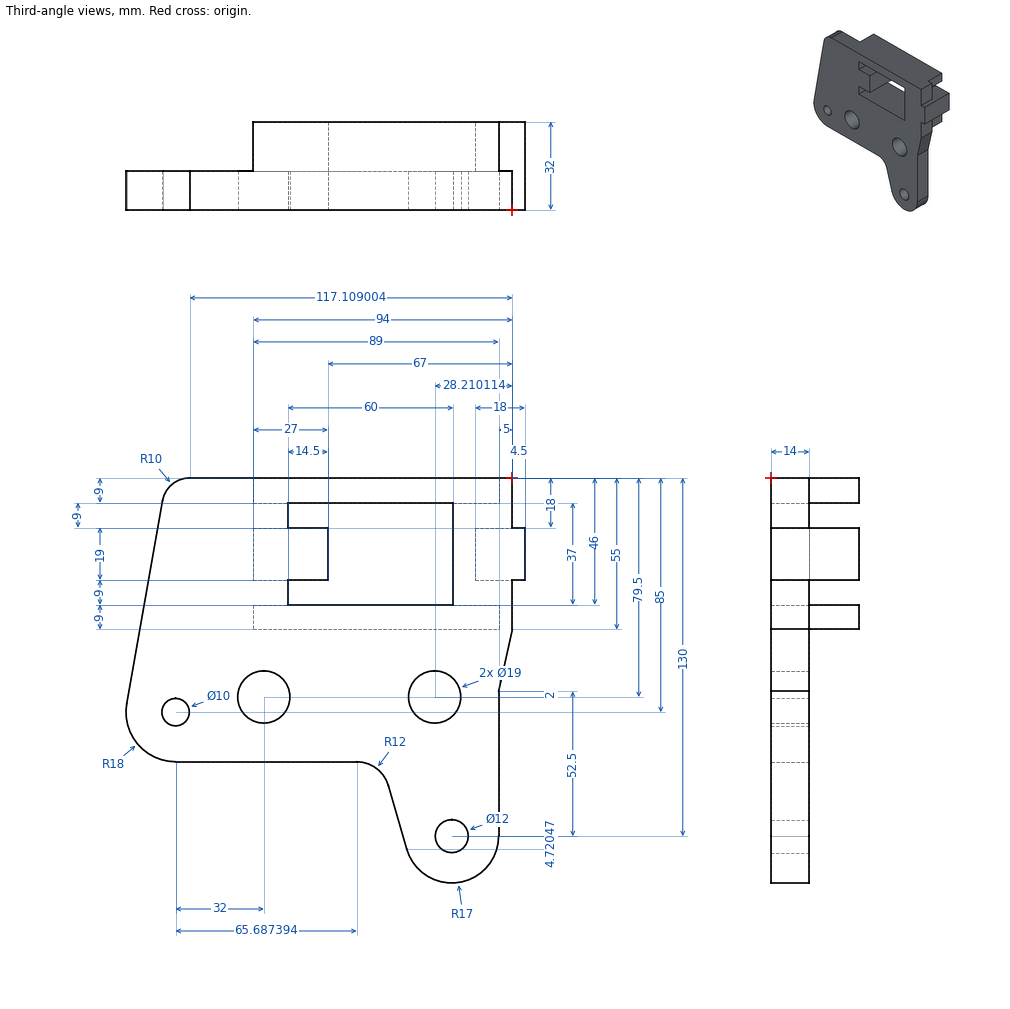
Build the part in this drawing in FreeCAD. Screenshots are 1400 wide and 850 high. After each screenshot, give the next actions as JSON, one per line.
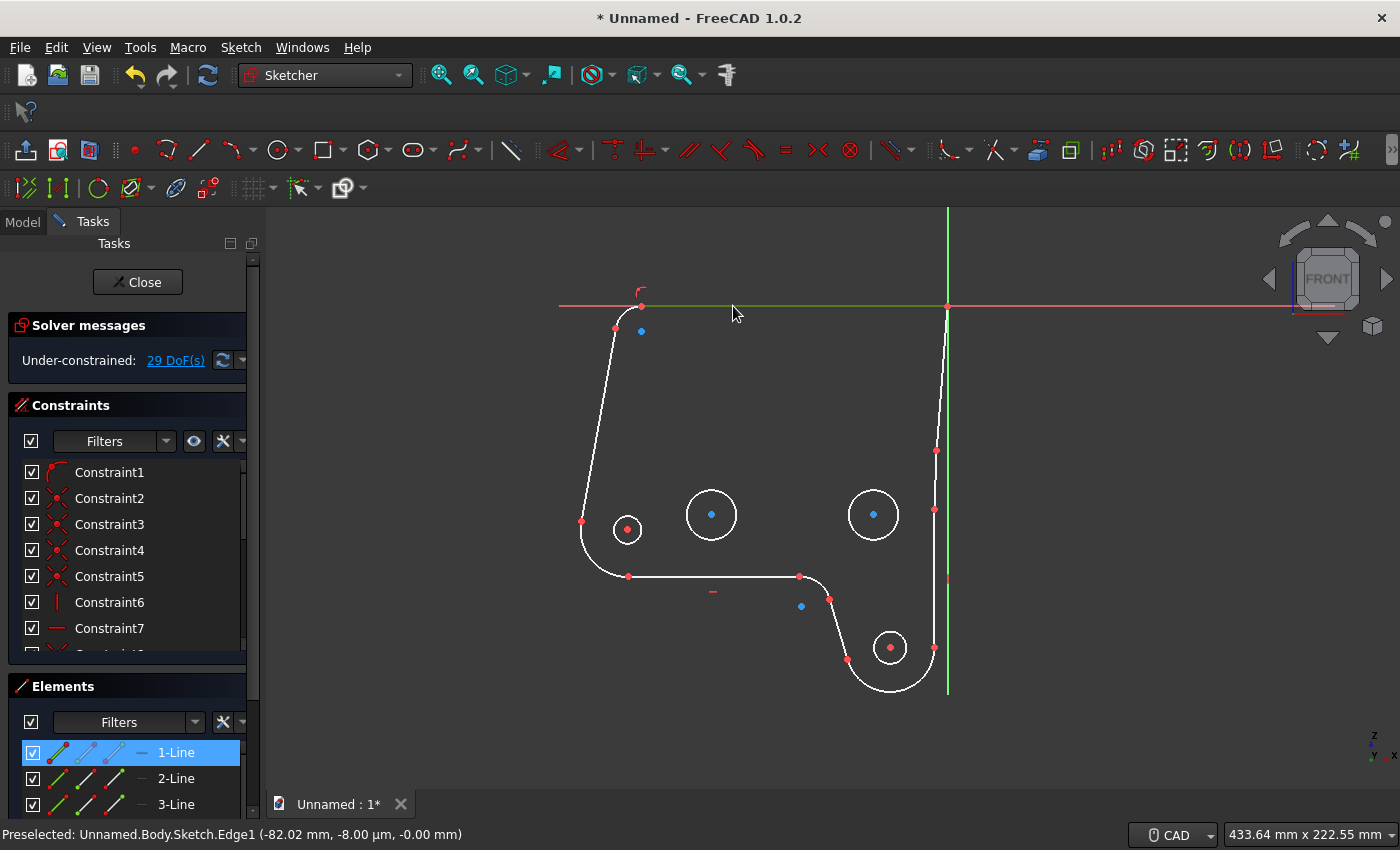
{"action": "scroll", "coordinate": [630, 309], "scroll_direction": "up", "scroll_amount": 2}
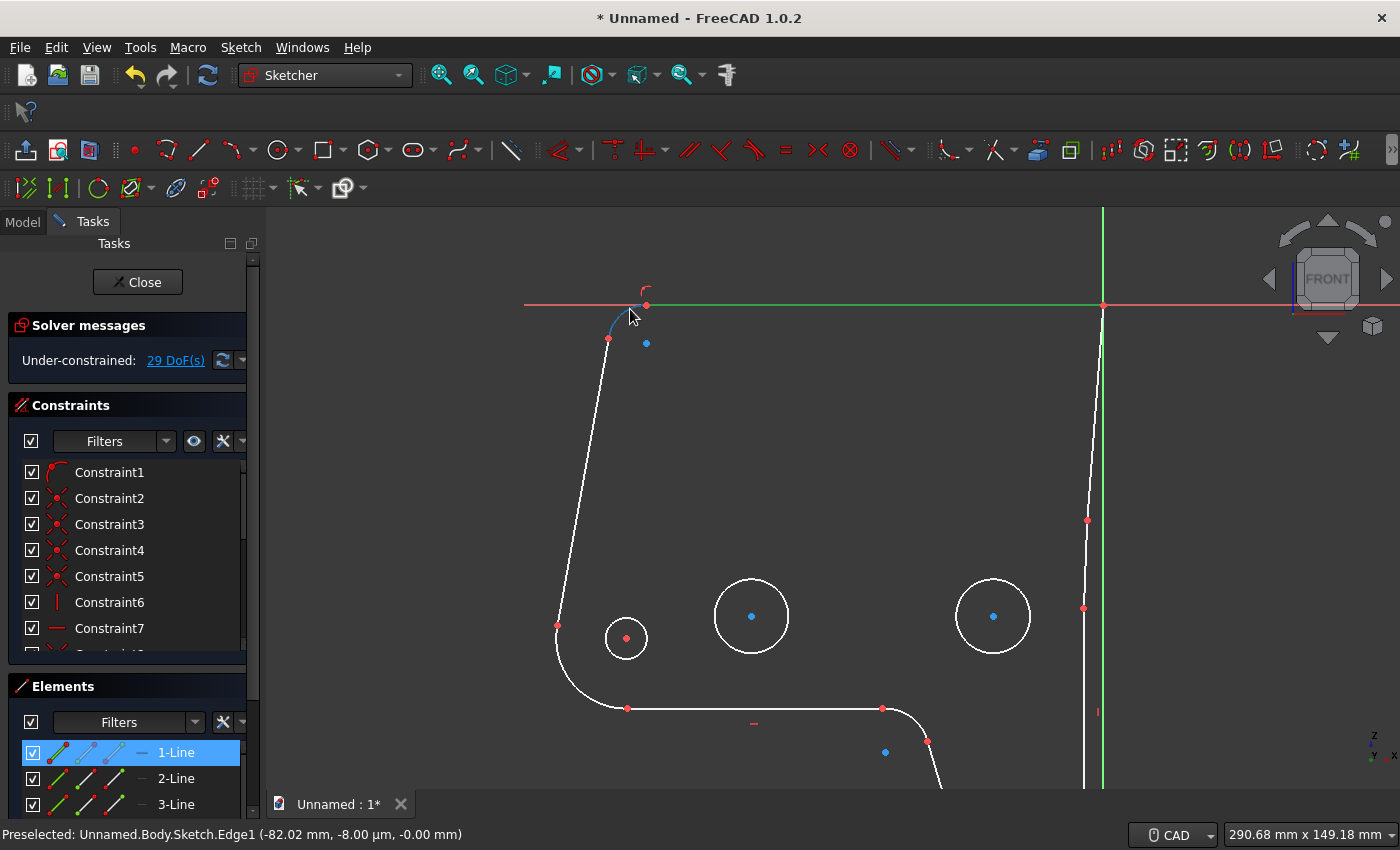
{"action": "left_click", "coordinate": [630, 309]}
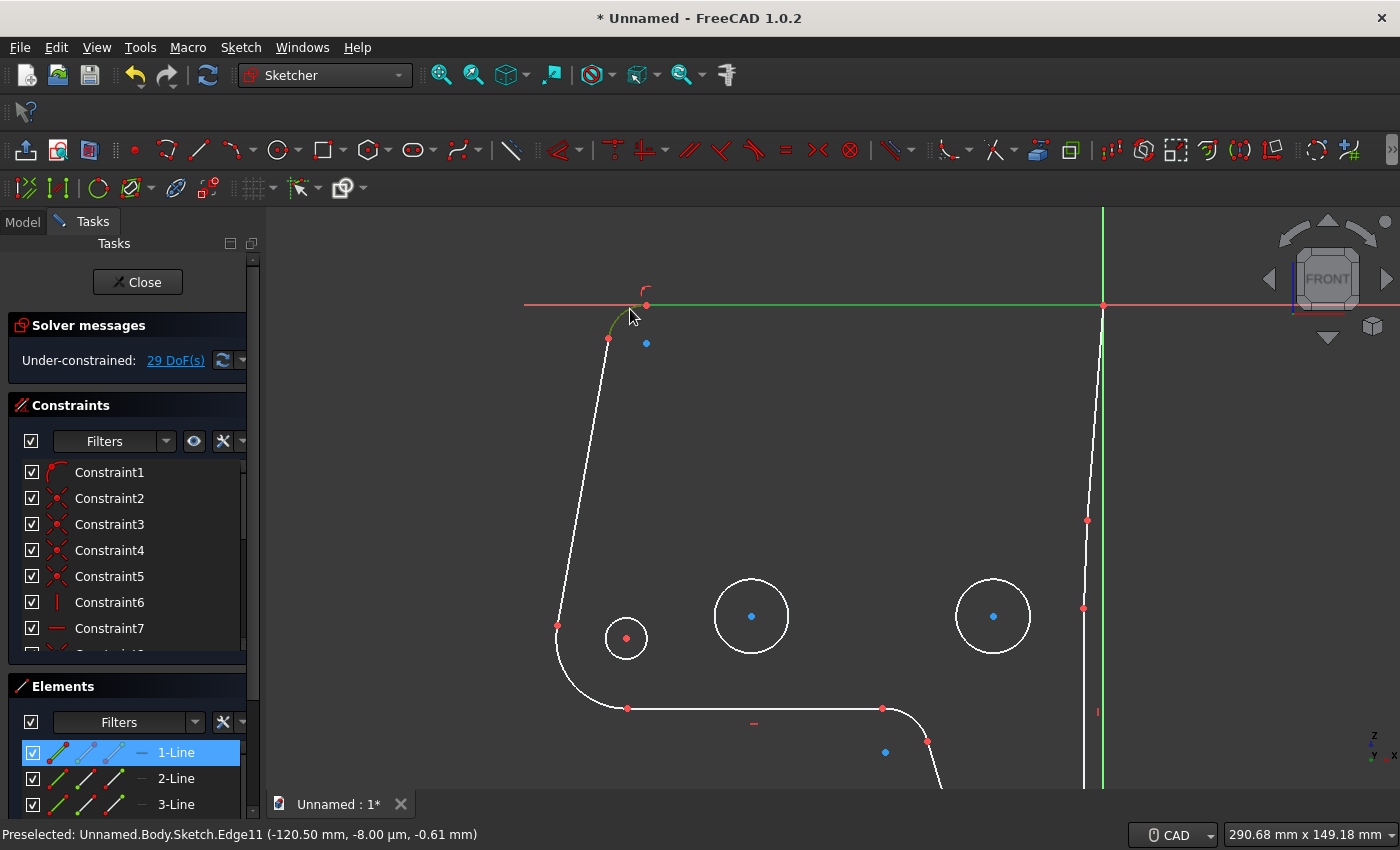
{"action": "left_click", "coordinate": [754, 150]}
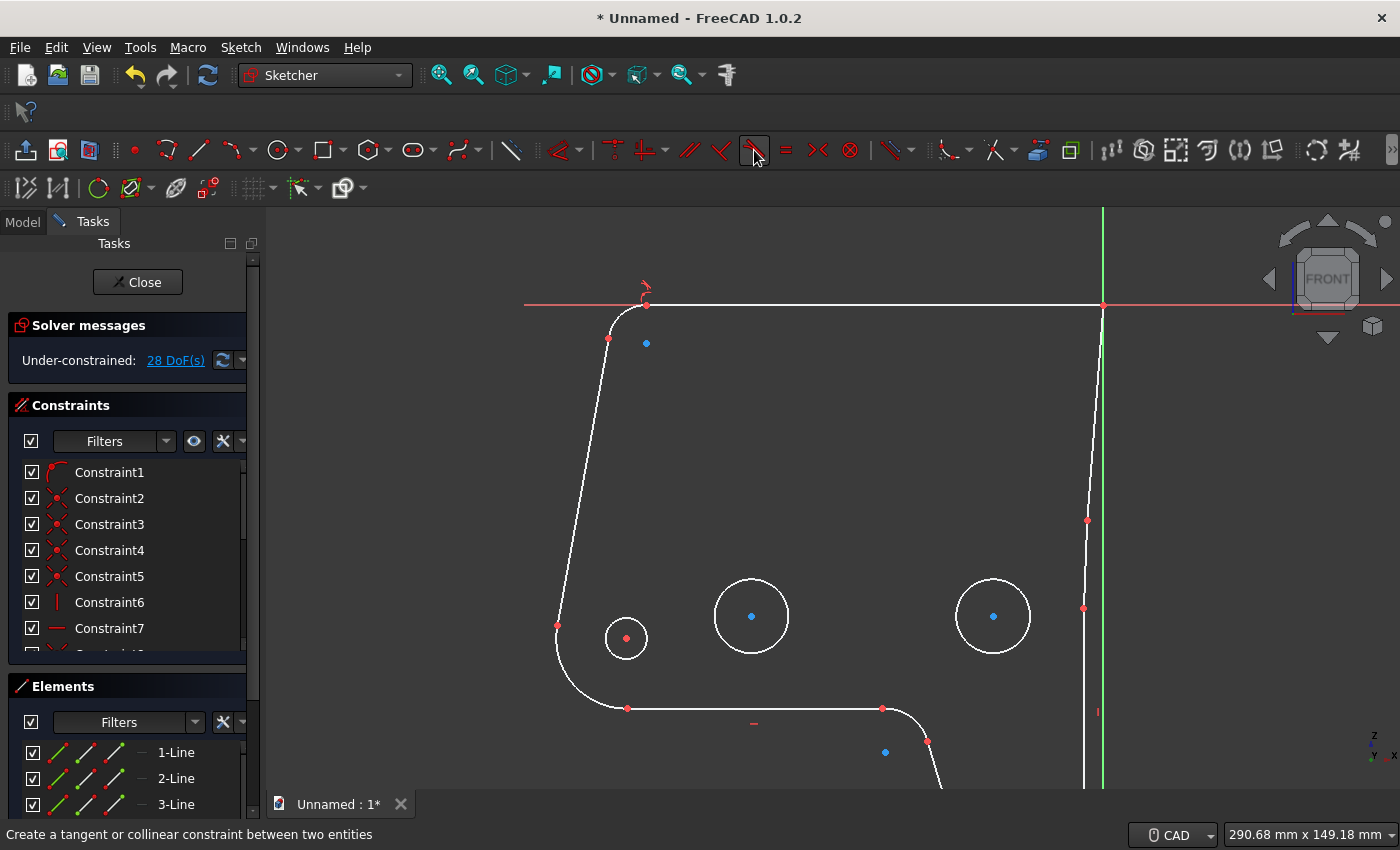
{"action": "left_click", "coordinate": [1084, 670]}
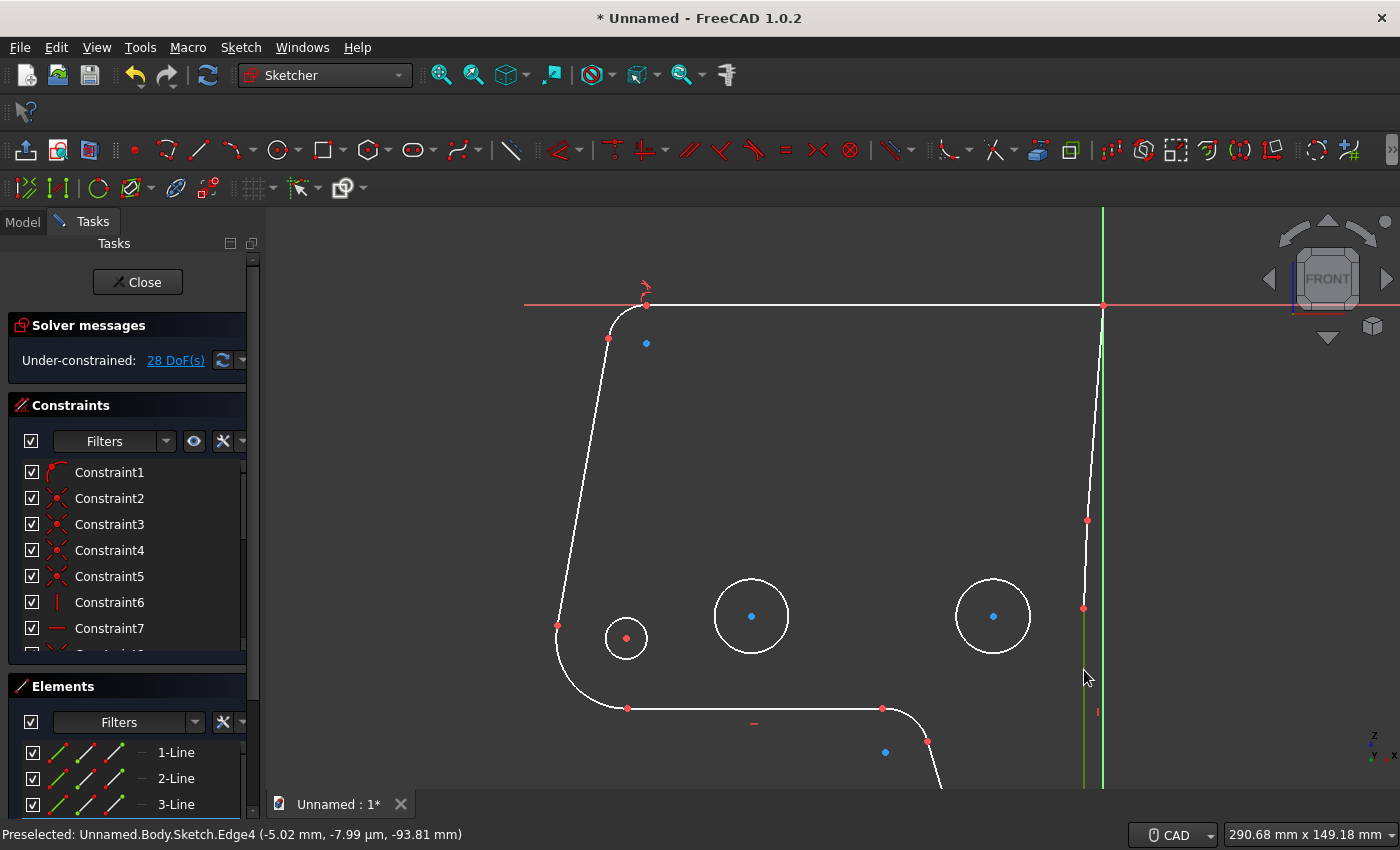
{"action": "scroll", "coordinate": [630, 308], "scroll_direction": "down", "scroll_amount": 2}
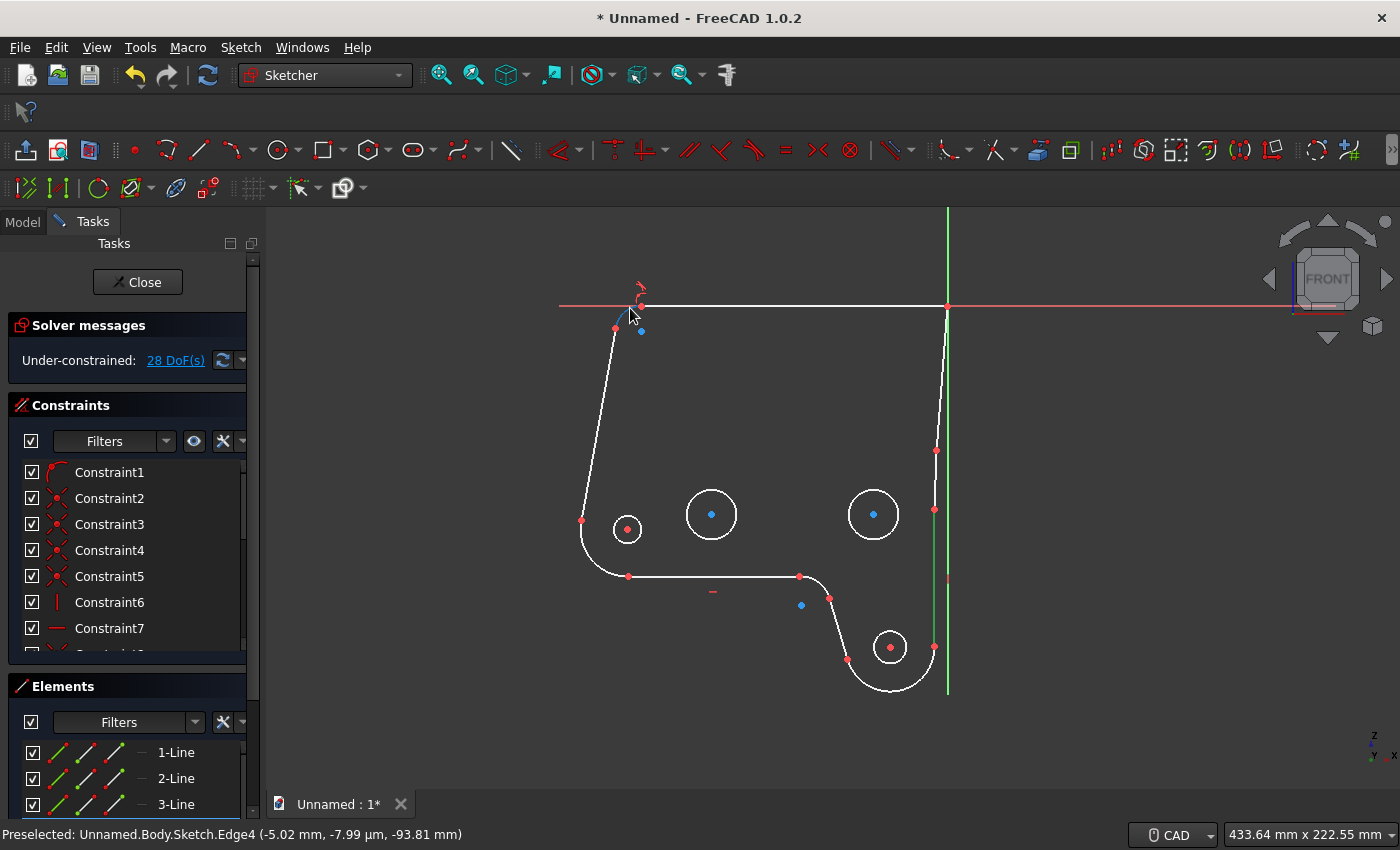
{"action": "left_click", "coordinate": [872, 687]}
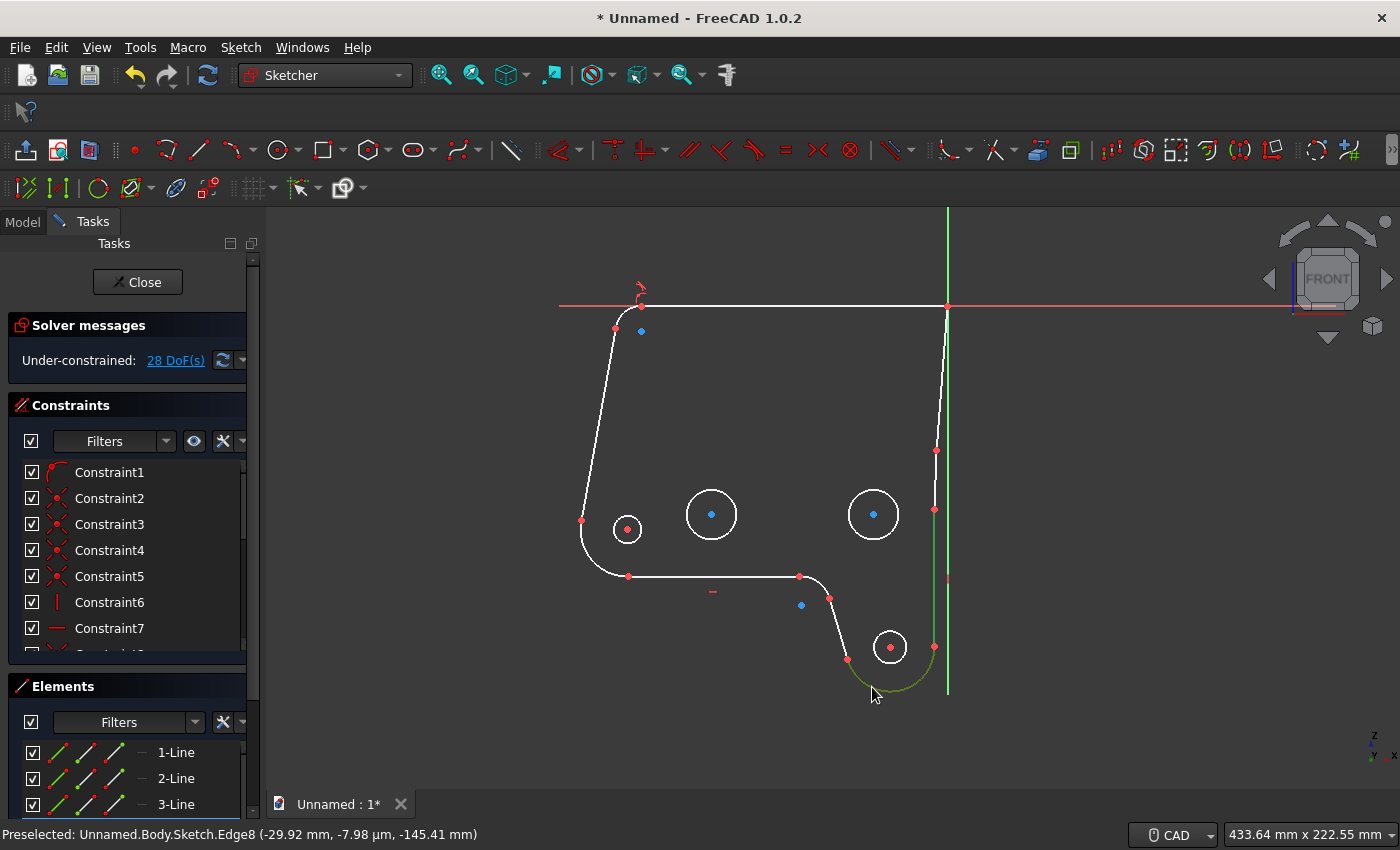
{"action": "left_click", "coordinate": [754, 150]}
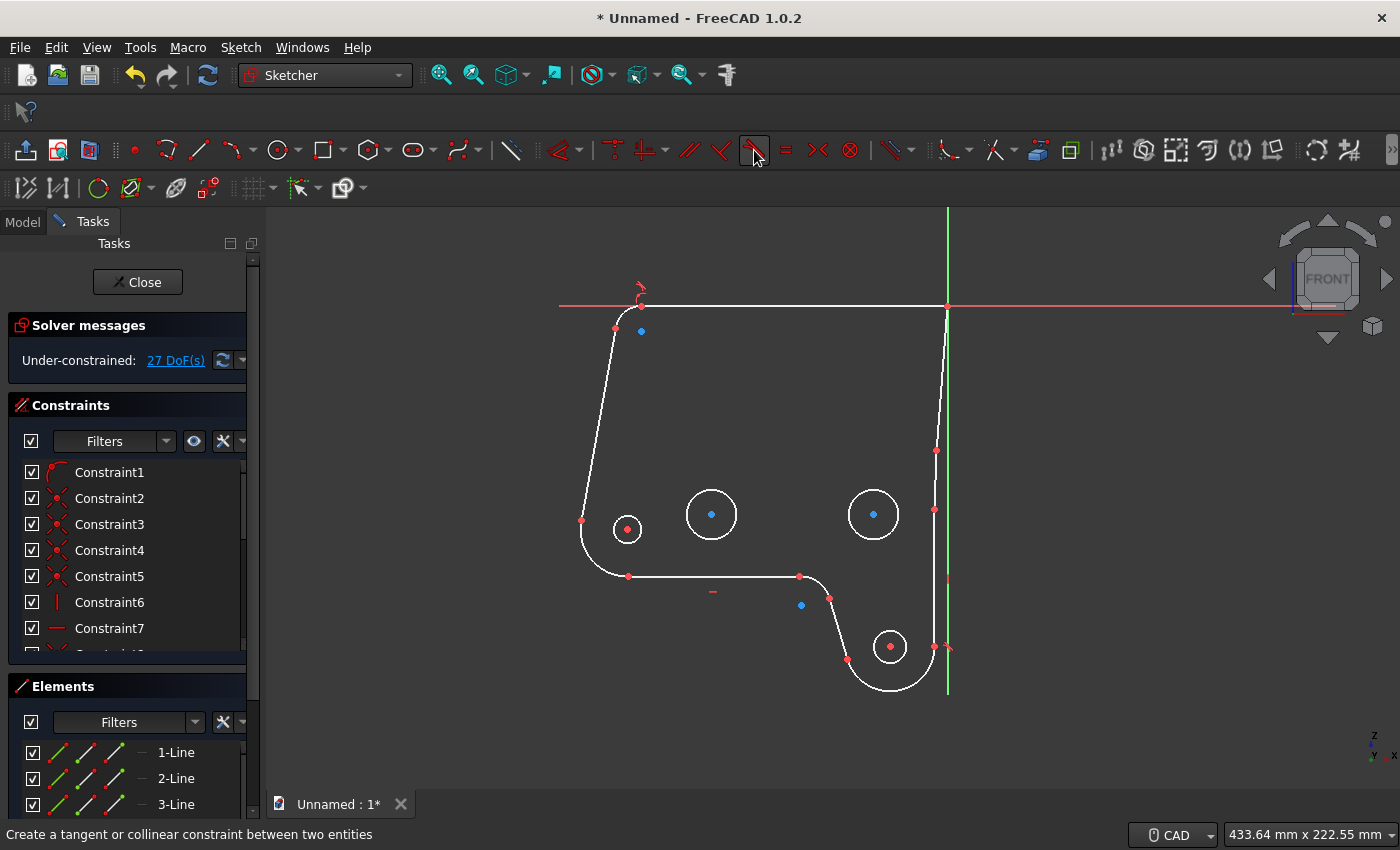
{"action": "left_click", "coordinate": [842, 641]}